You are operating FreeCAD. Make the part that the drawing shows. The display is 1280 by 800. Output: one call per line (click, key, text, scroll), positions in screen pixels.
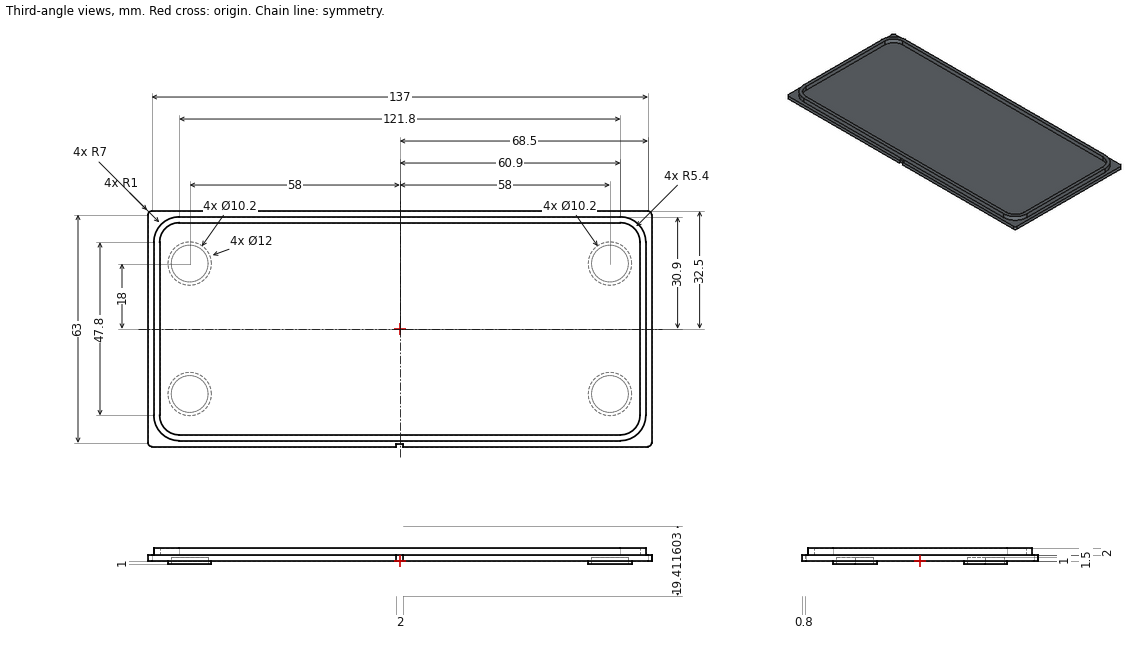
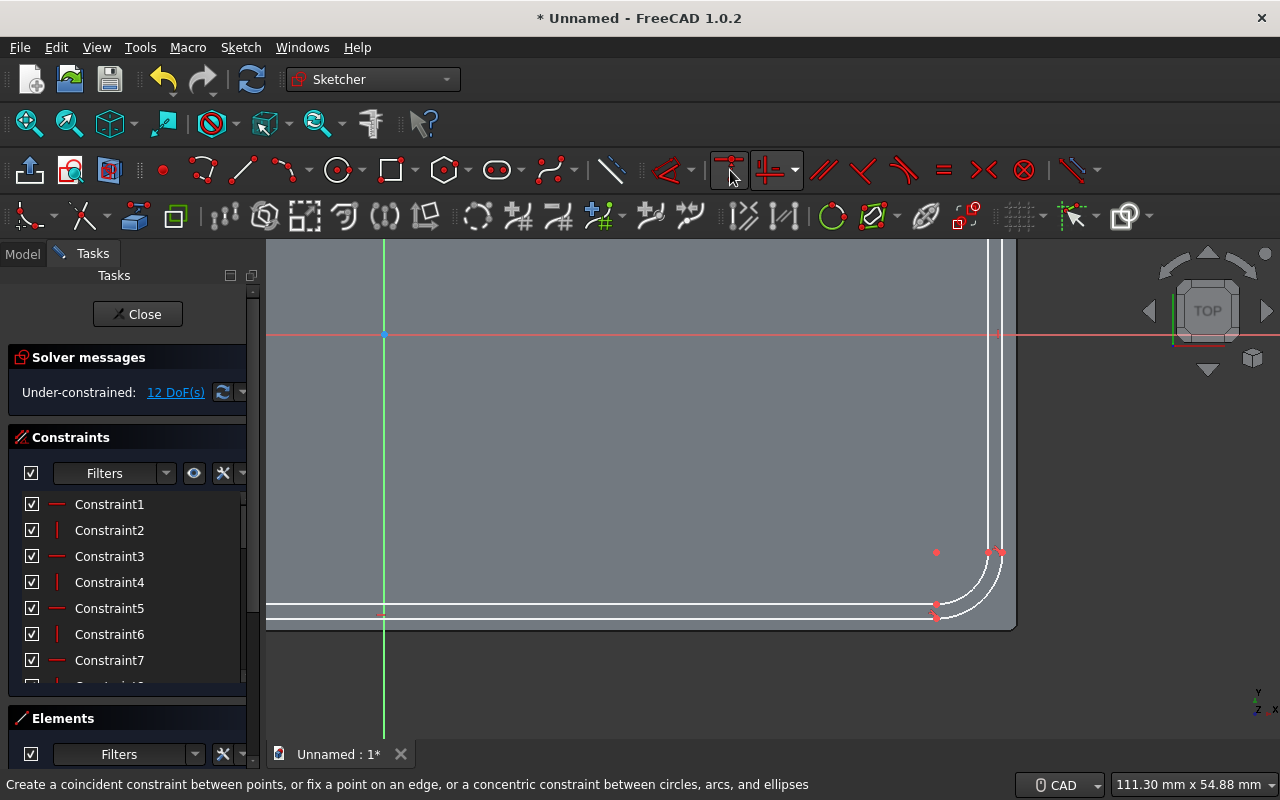
scroll(966, 615, down, 4)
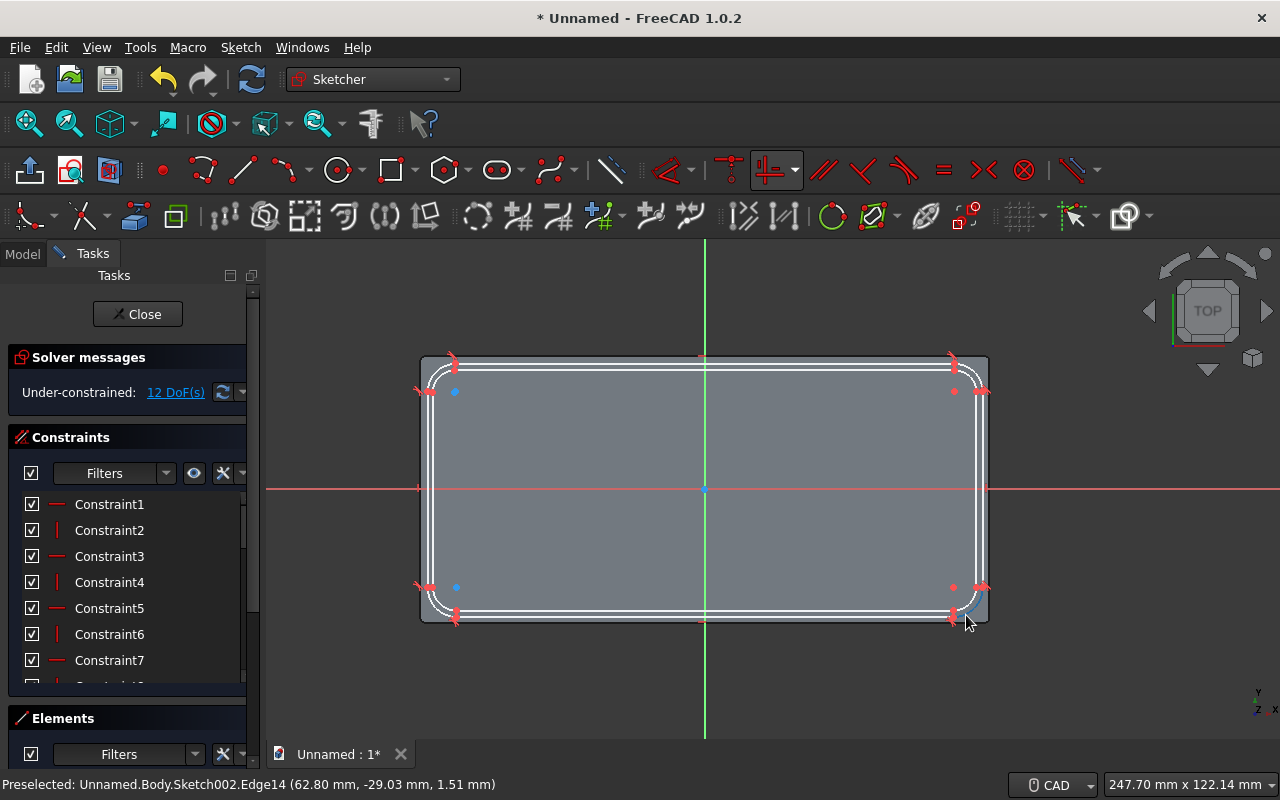
scroll(431, 601, up, 5)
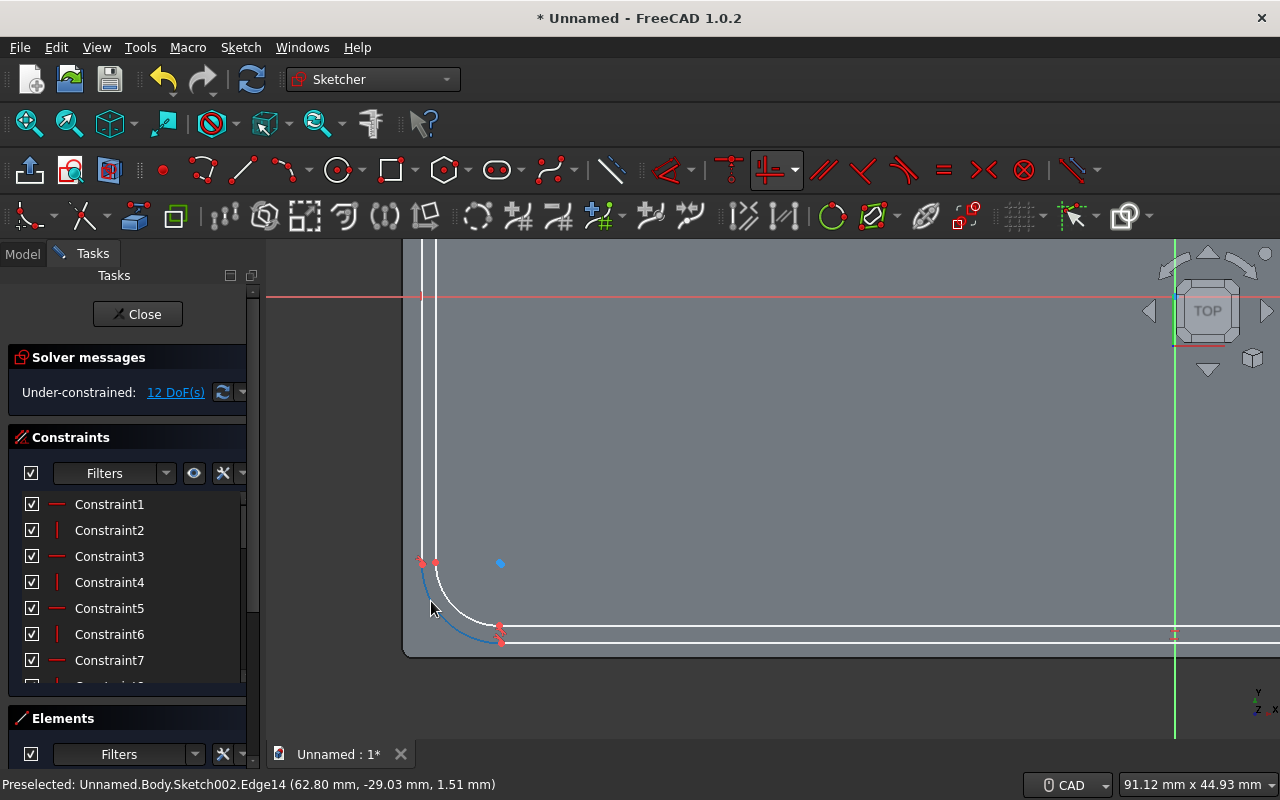
click(431, 600)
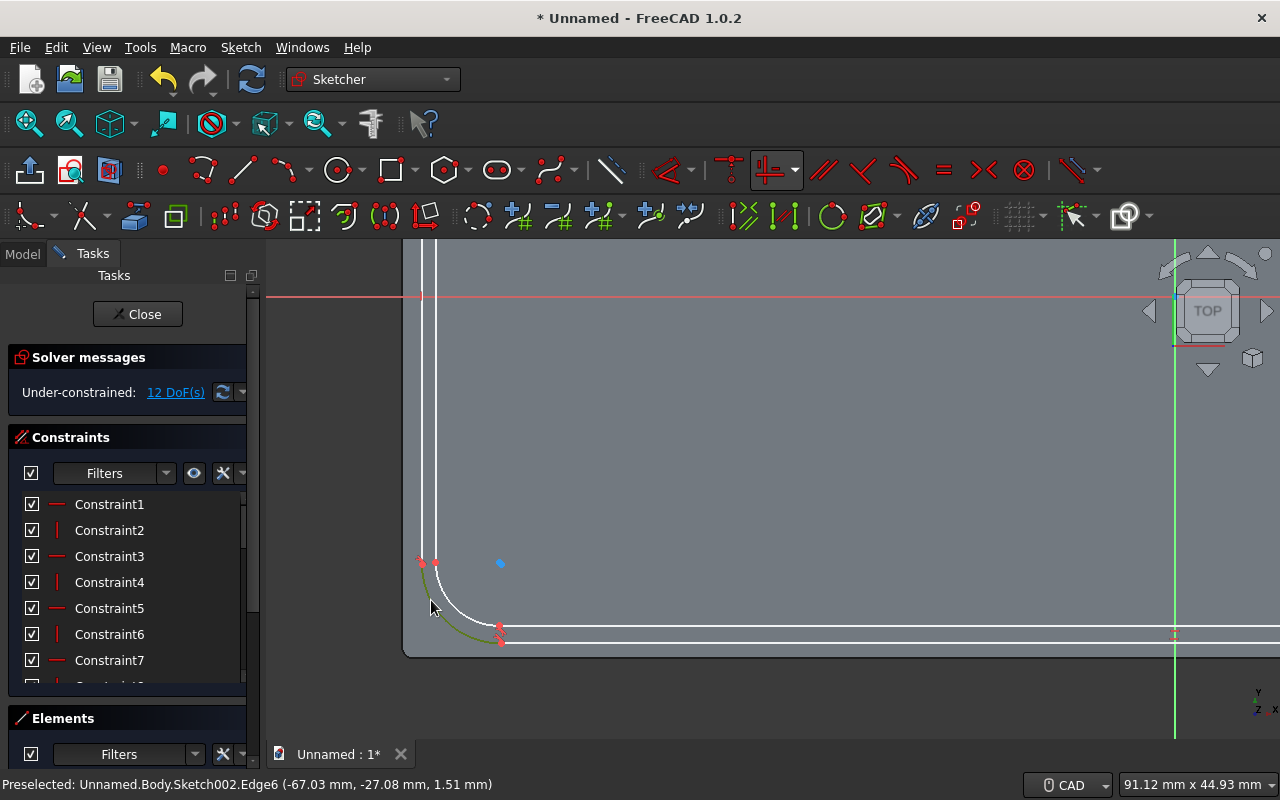
click(443, 591)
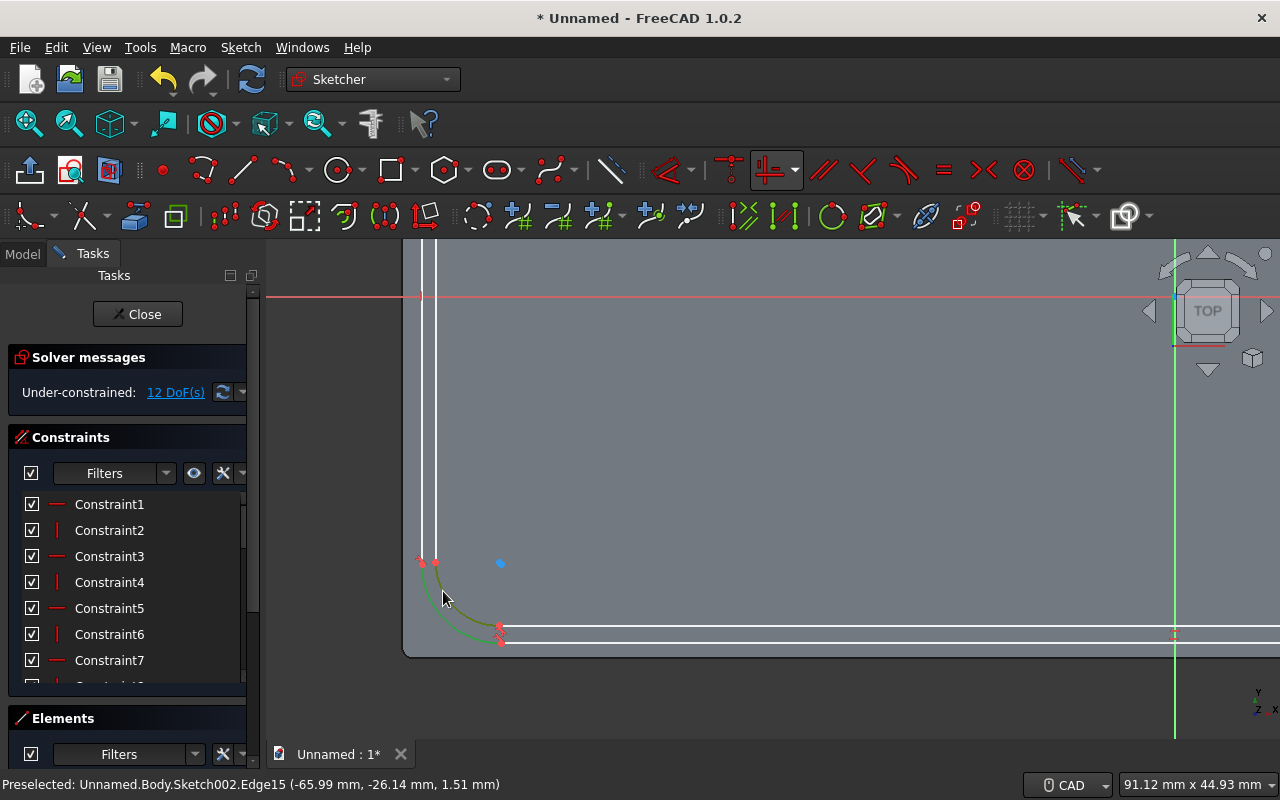
click(730, 170)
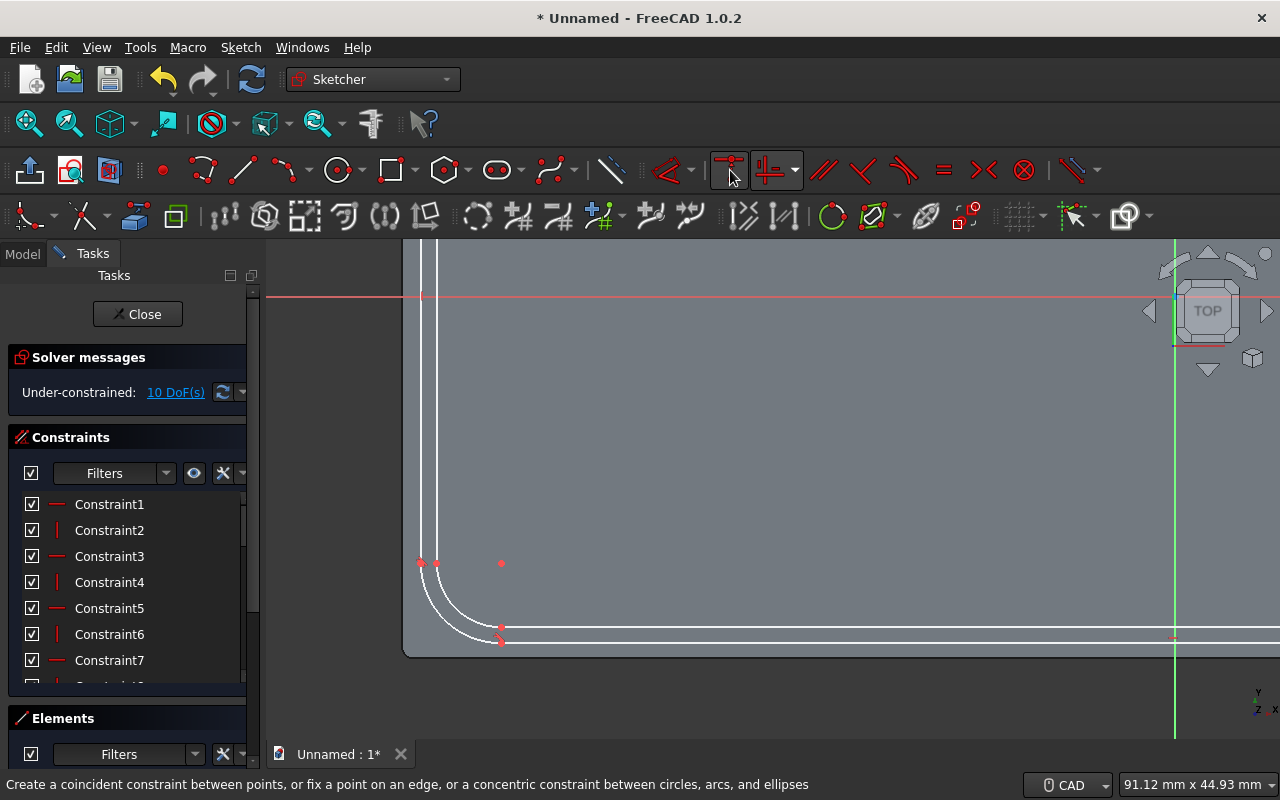
scroll(430, 601, down, 5)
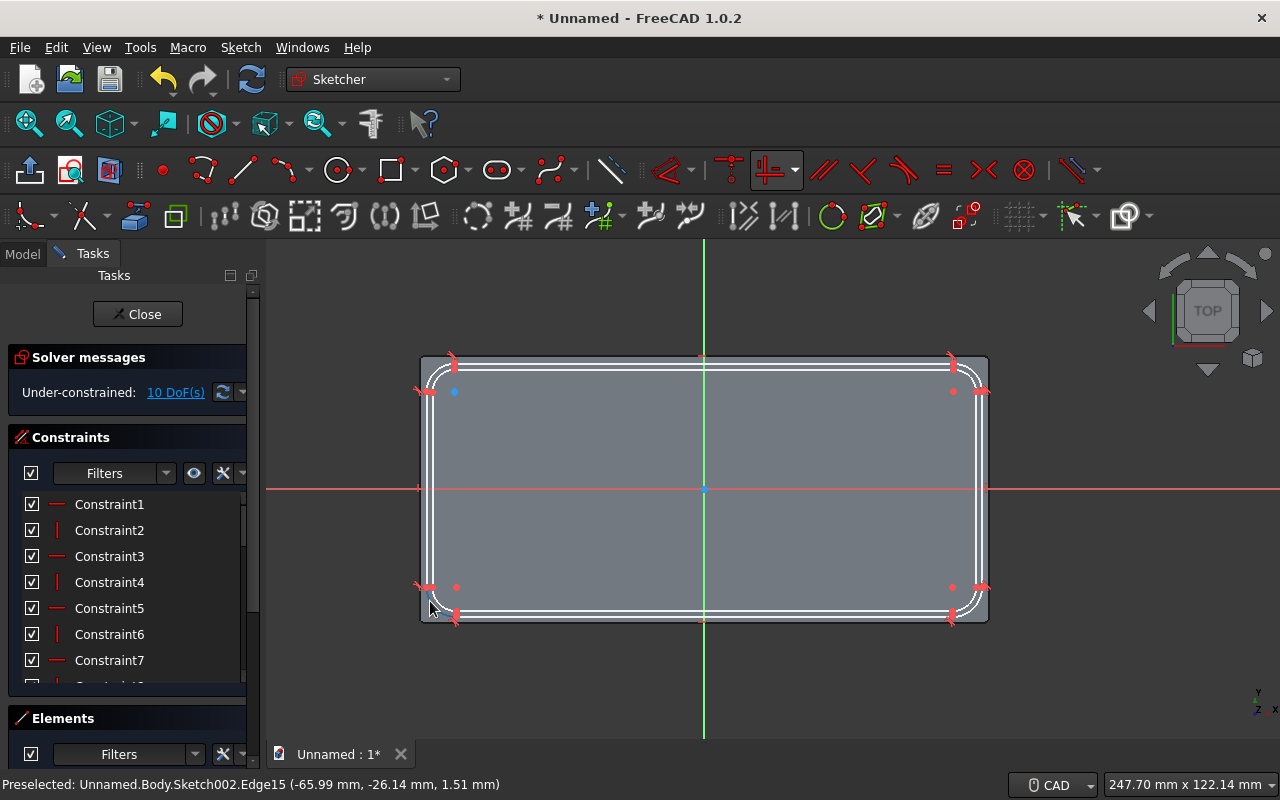
scroll(442, 367, up, 5)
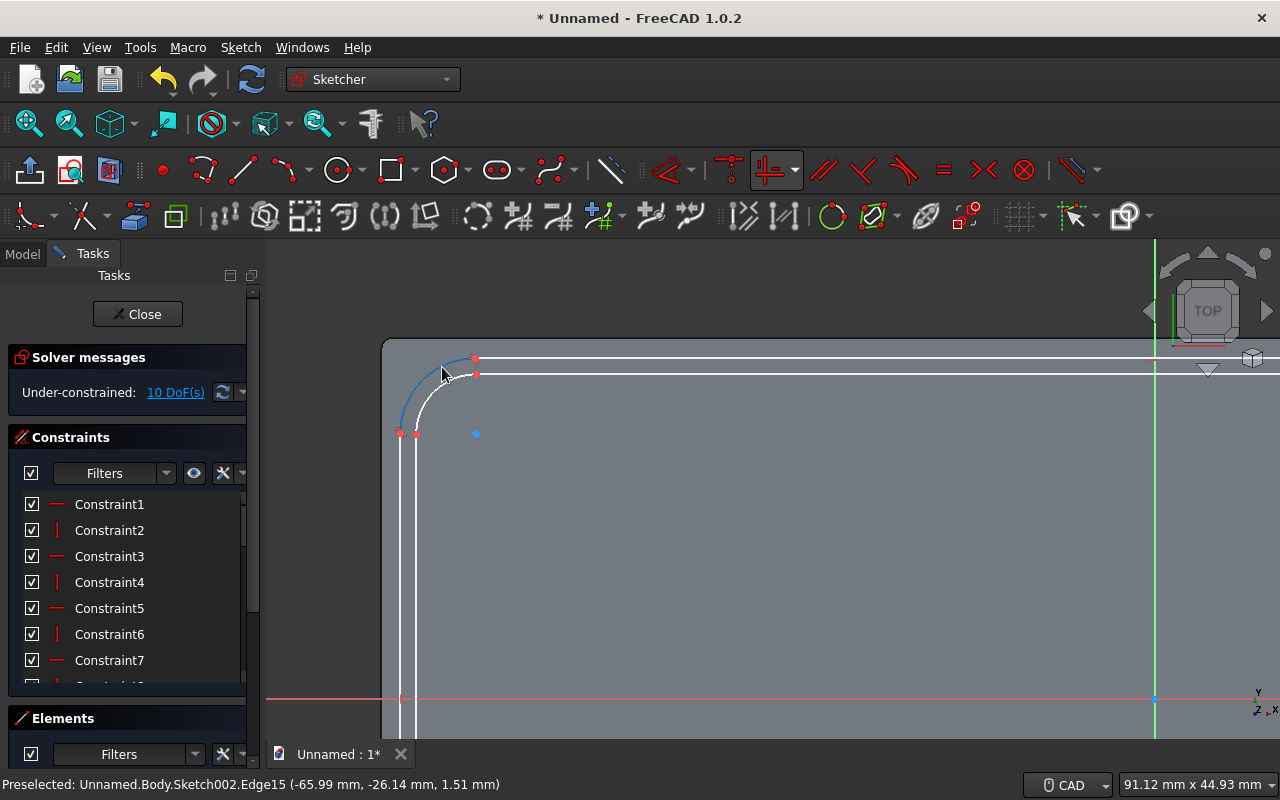
click(441, 367)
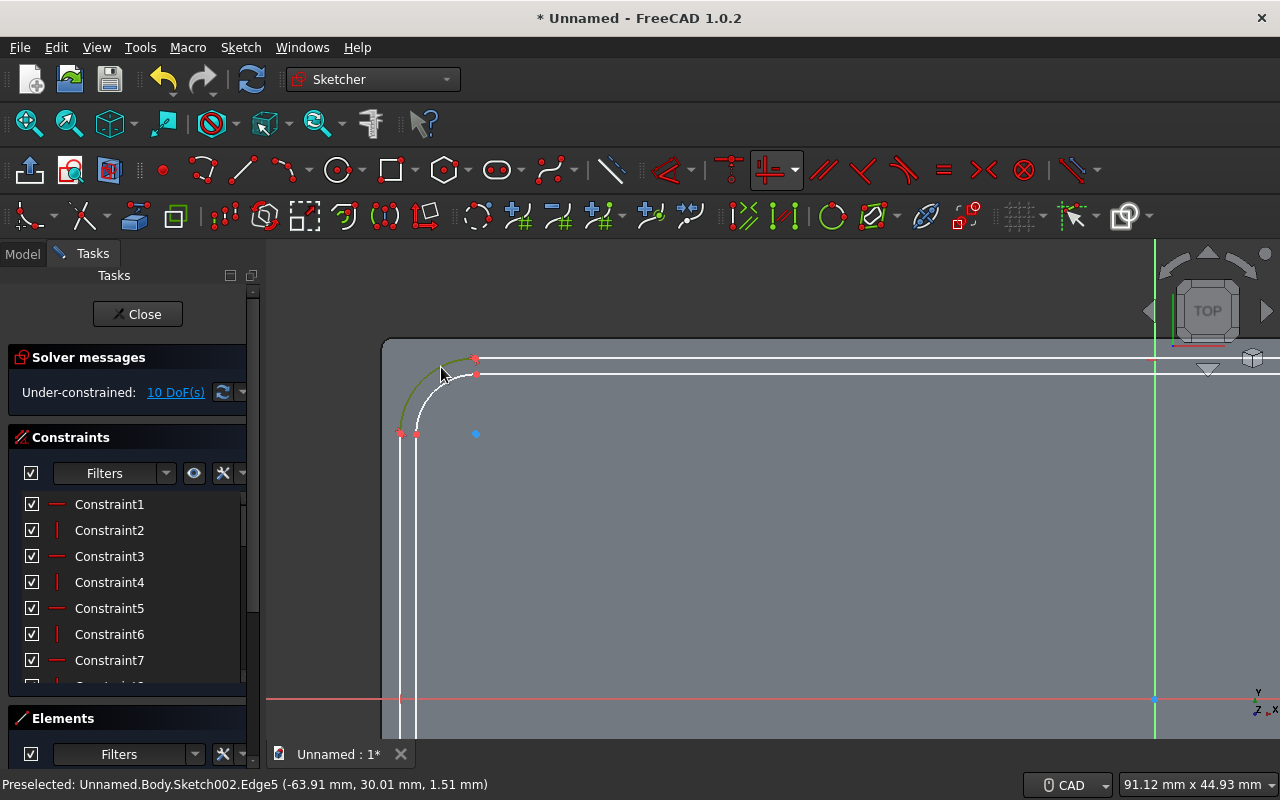
scroll(442, 366, down, 5)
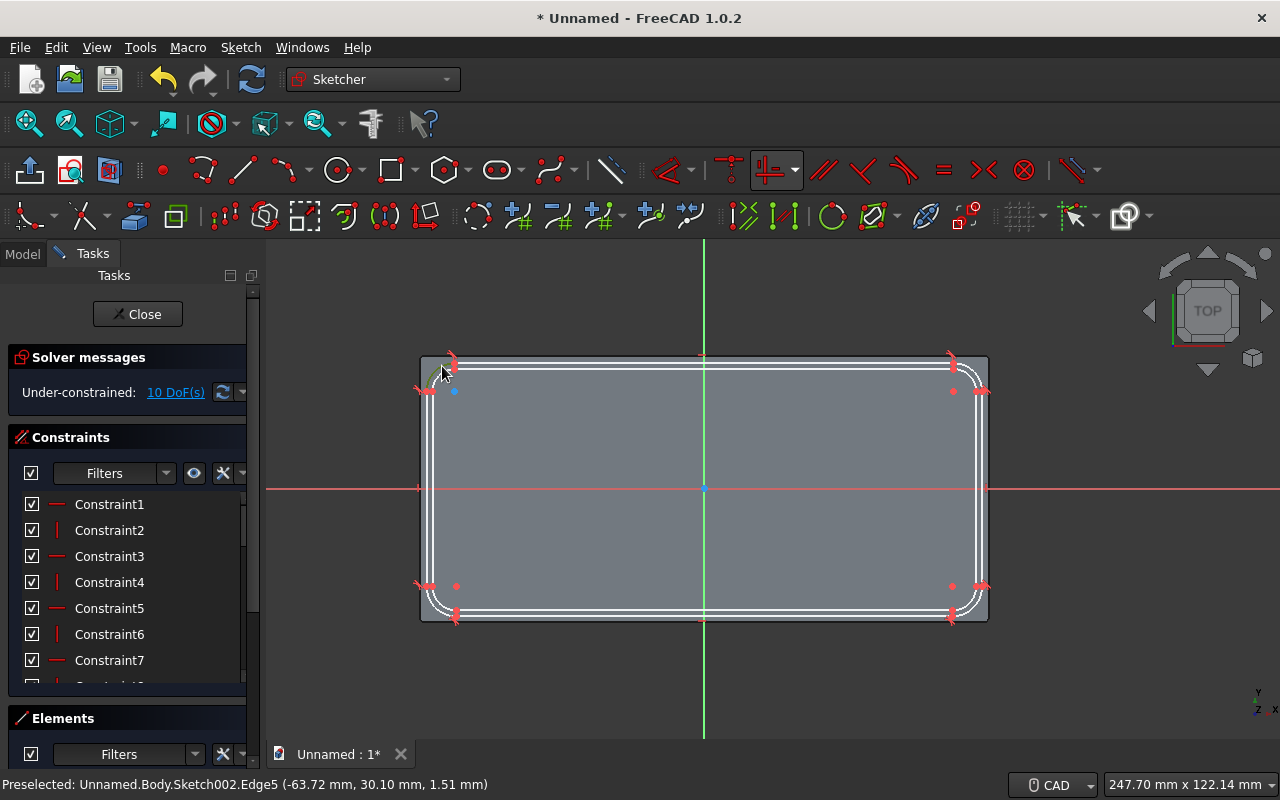
scroll(430, 600, up, 5)